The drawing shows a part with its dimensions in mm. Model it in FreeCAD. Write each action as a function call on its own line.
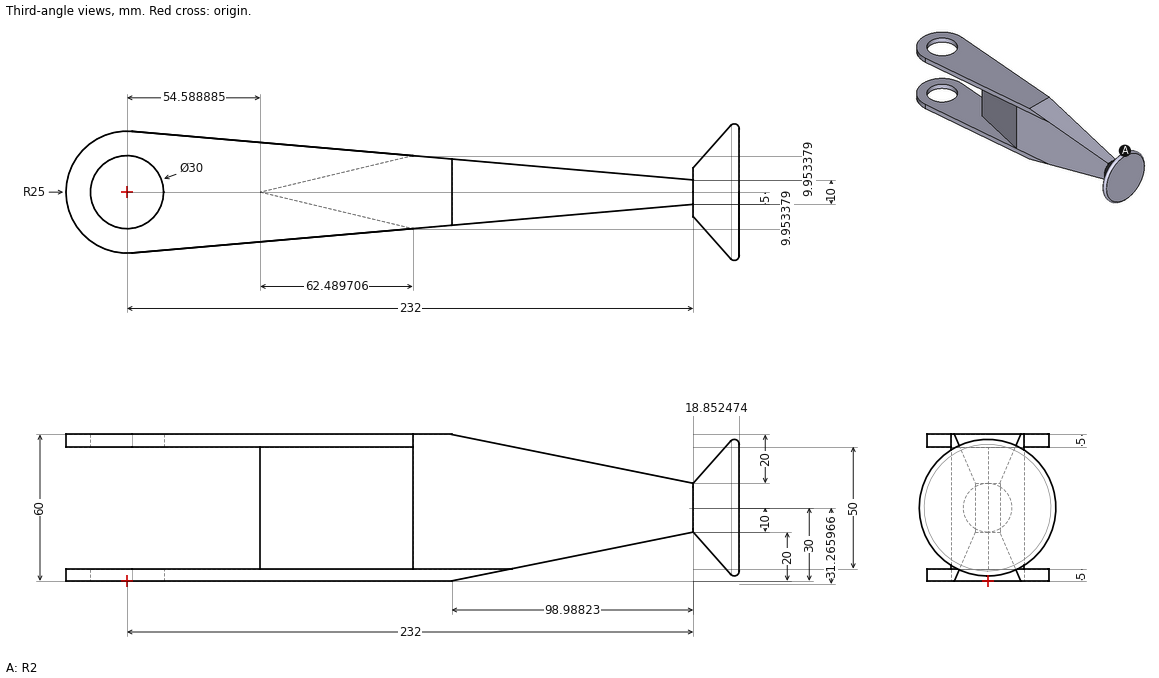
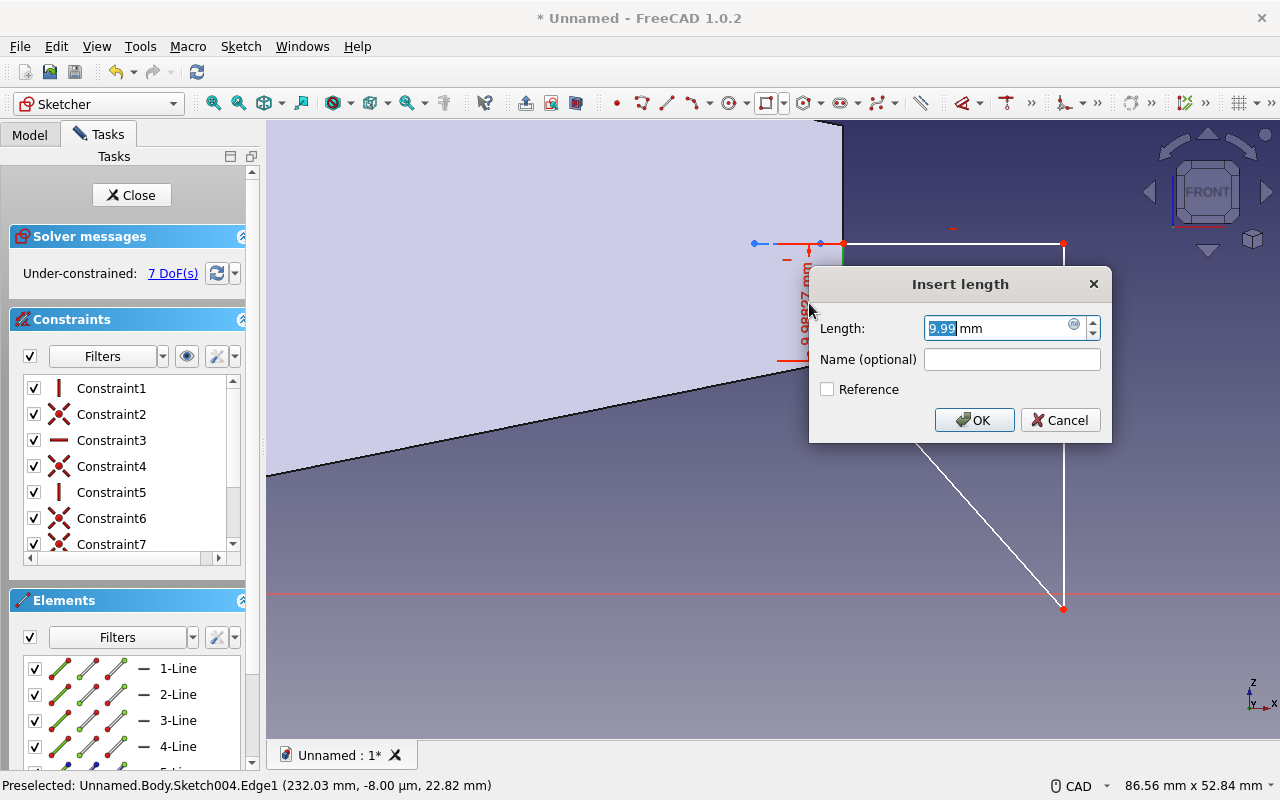
text(10)
key(Return)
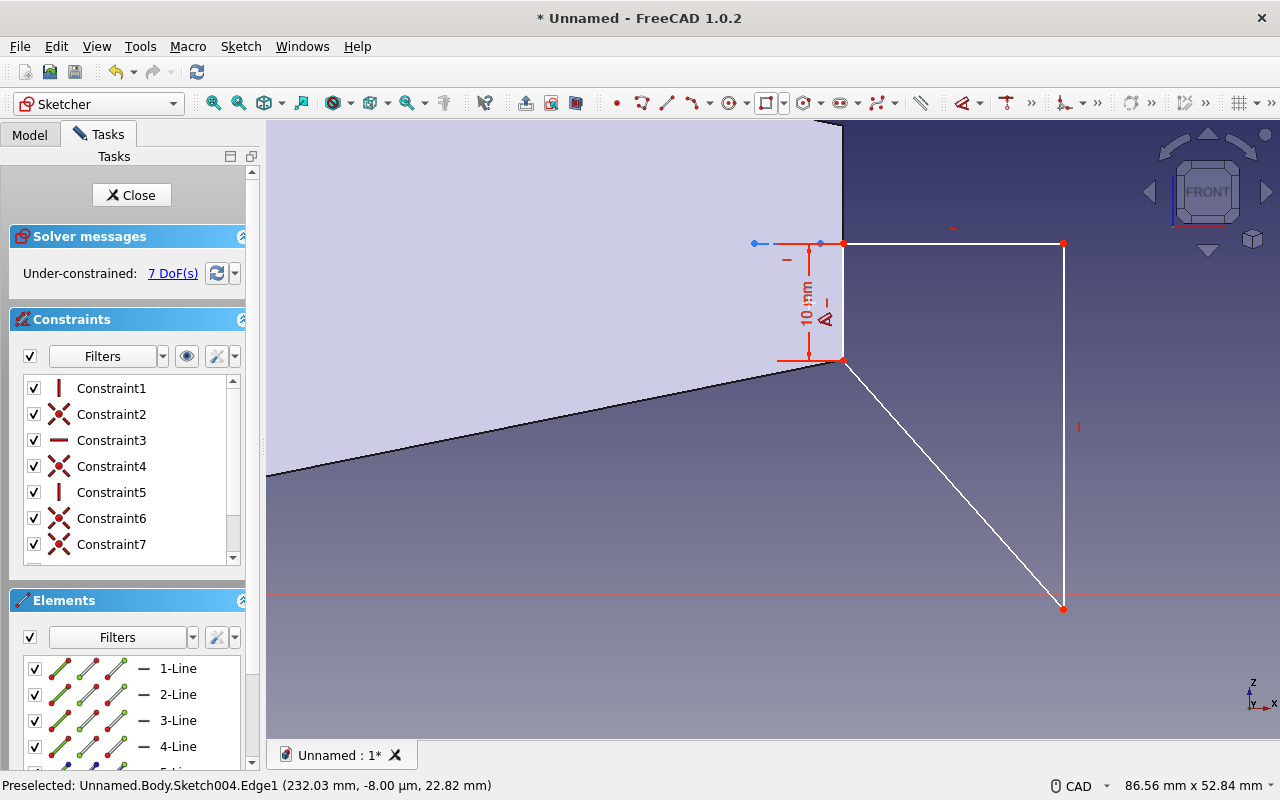
click(843, 361)
click(877, 478)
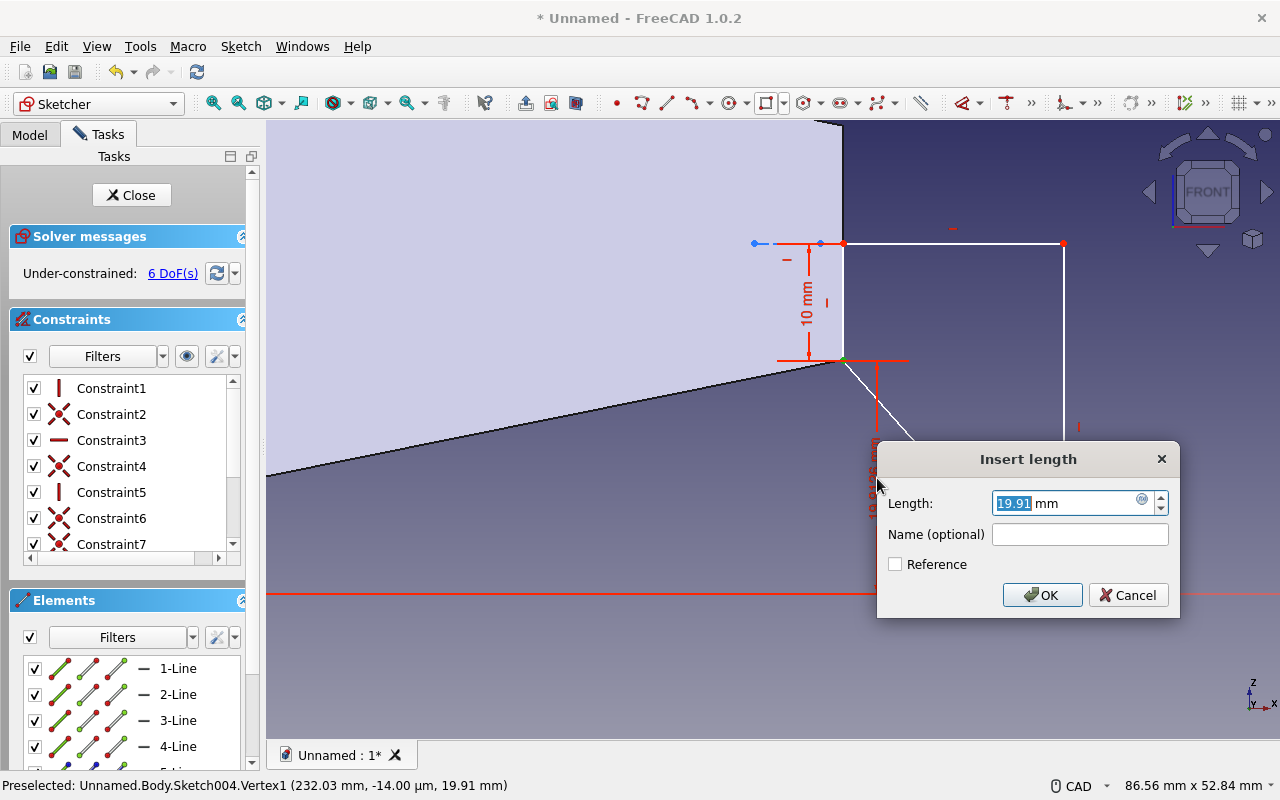
text(20)
key(Return)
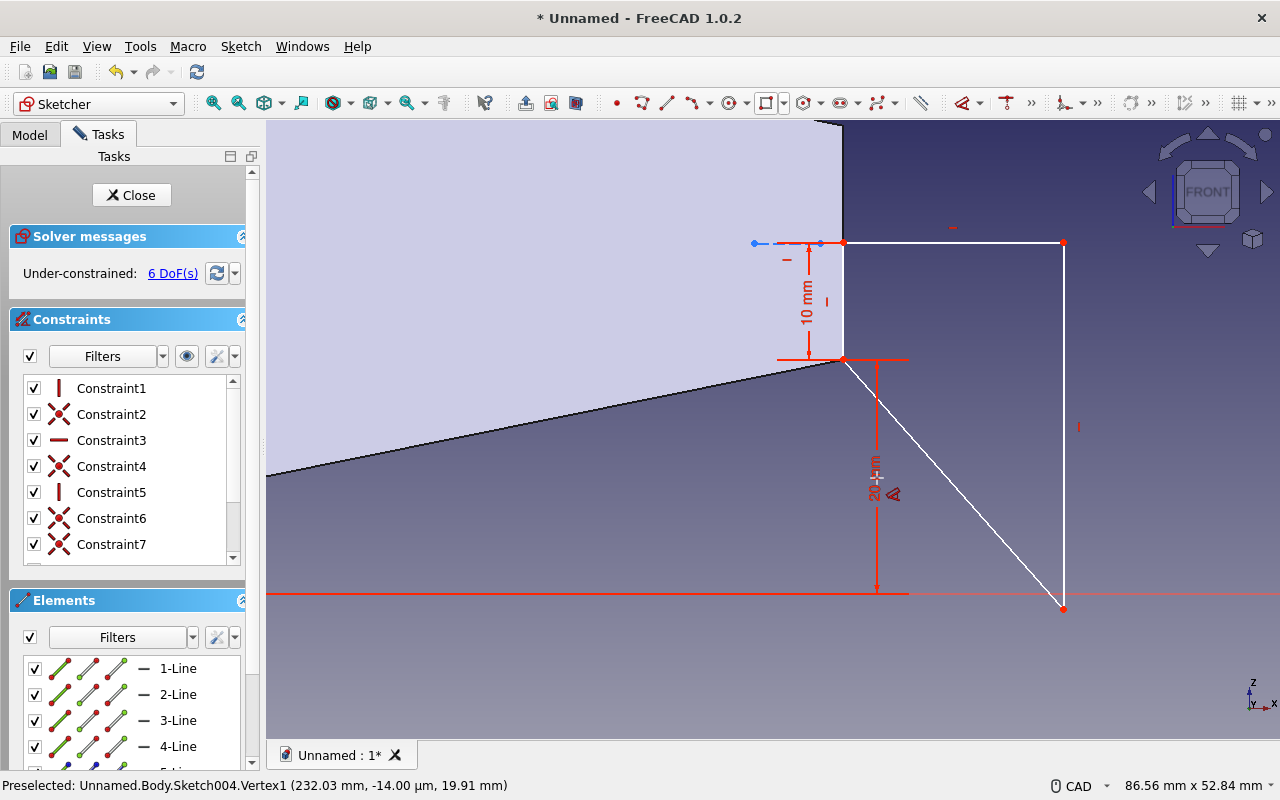
click(821, 244)
click(855, 419)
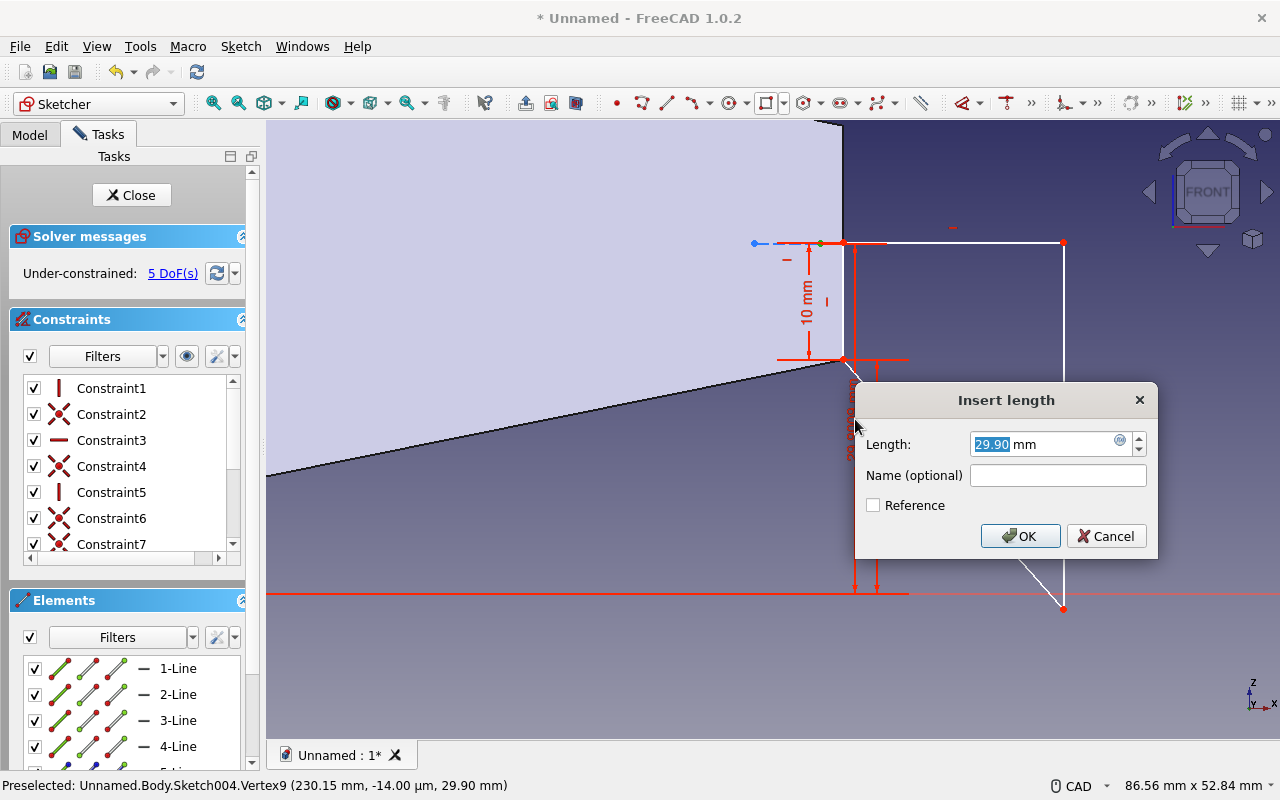
text(30)
key(Return)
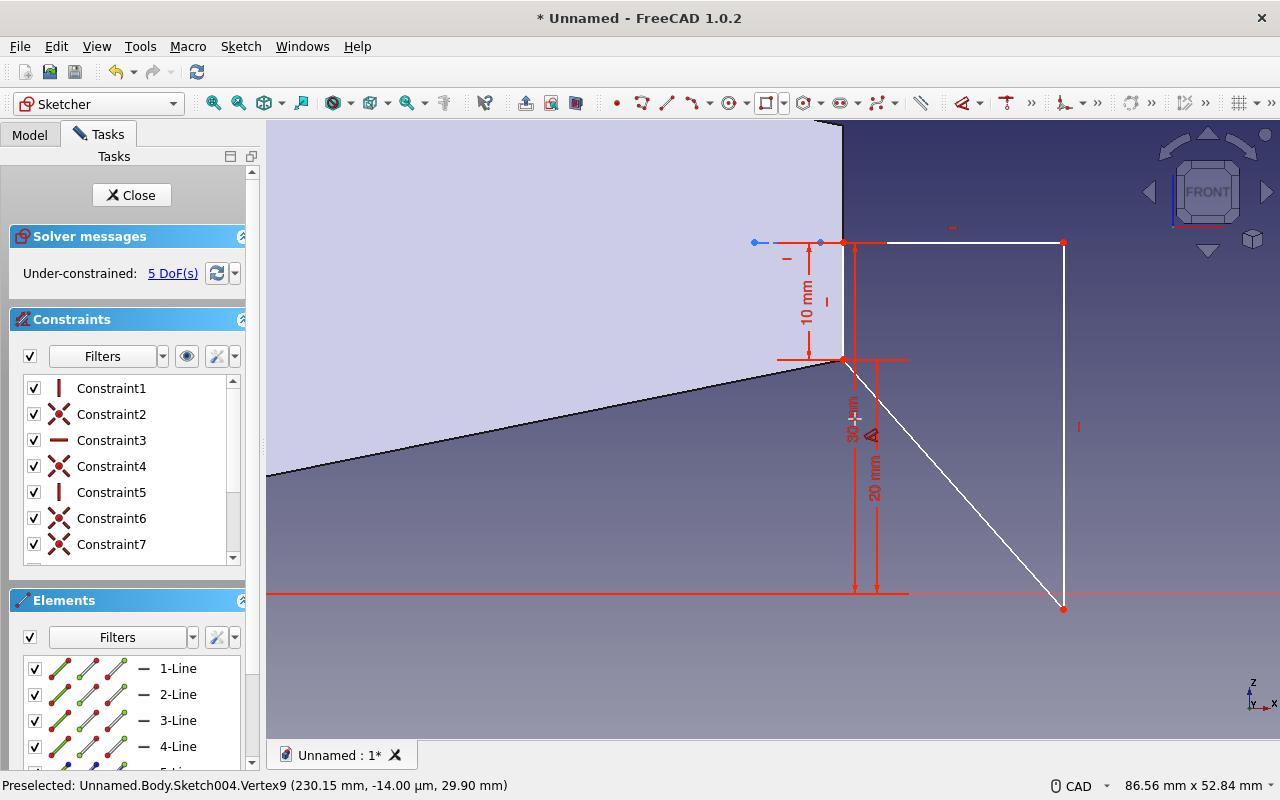
click(843, 360)
click(568, 628)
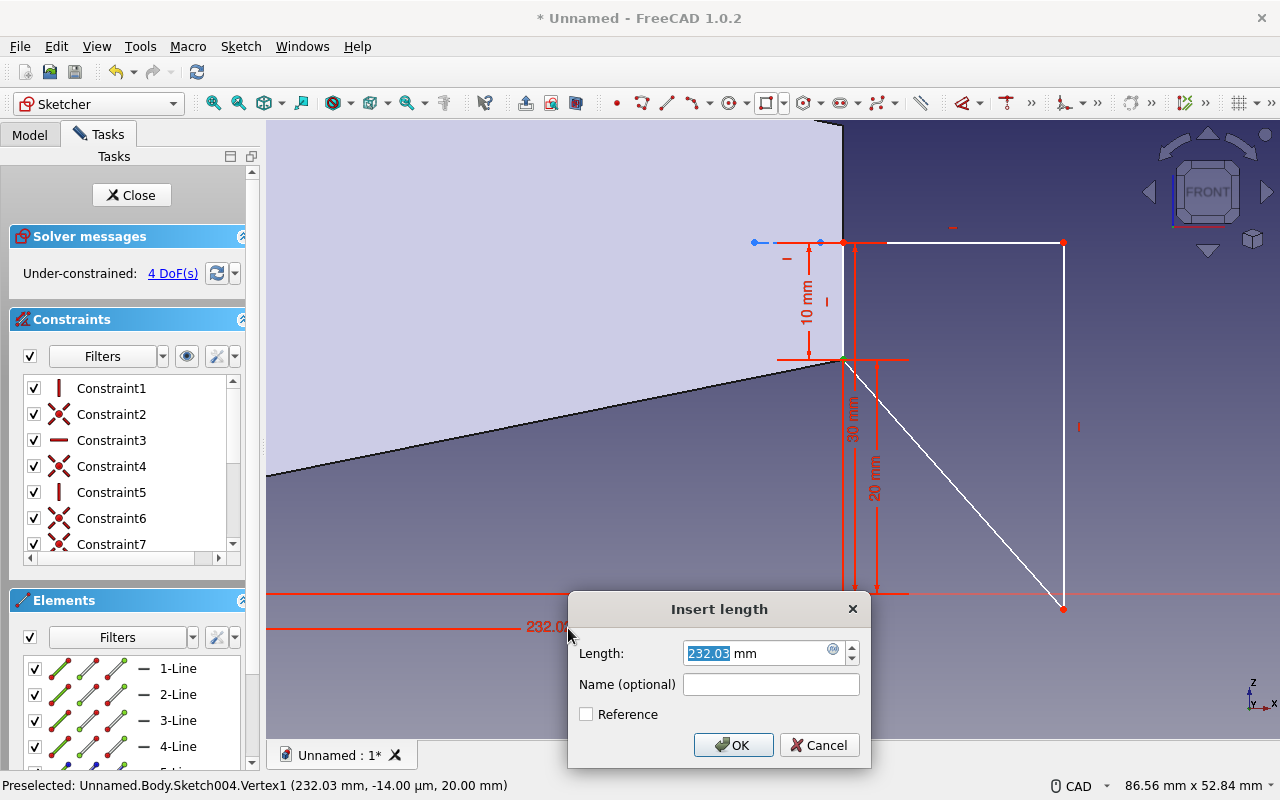
text(232)
key(Return)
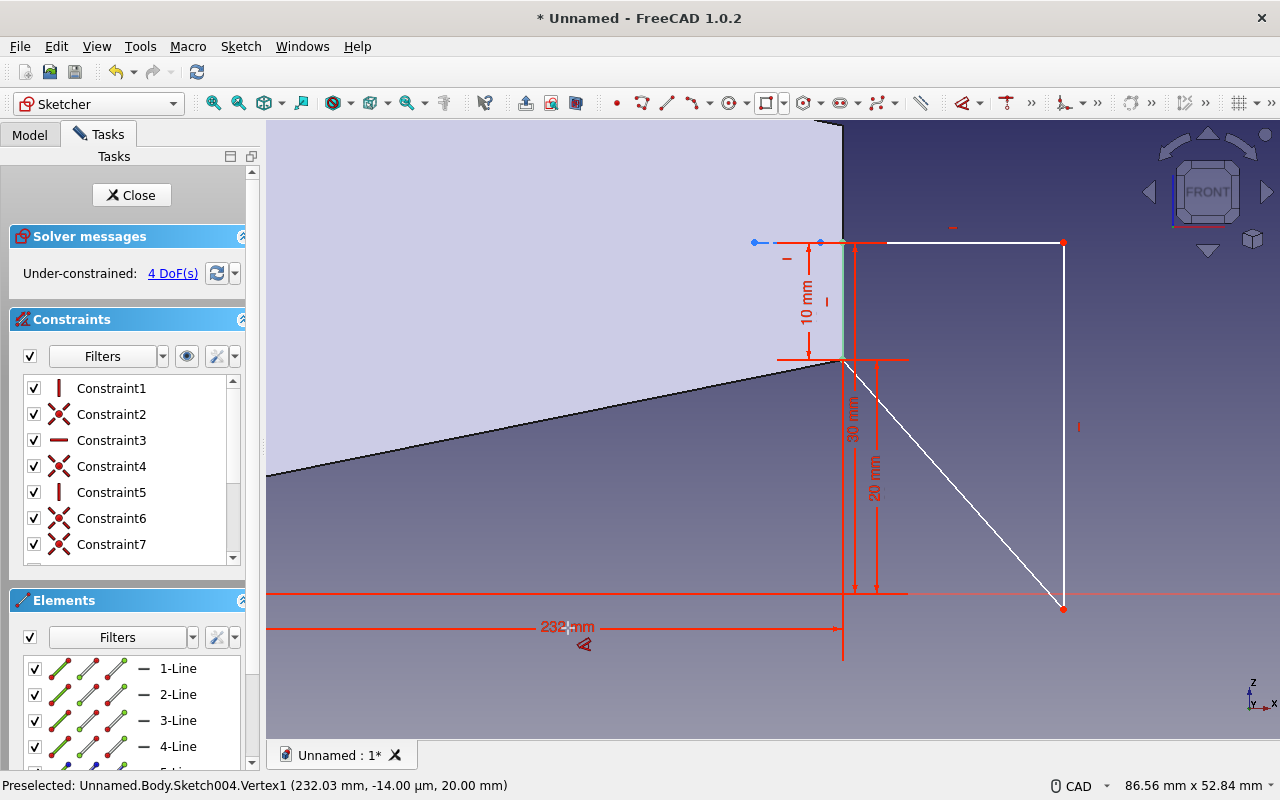
click(909, 243)
click(953, 209)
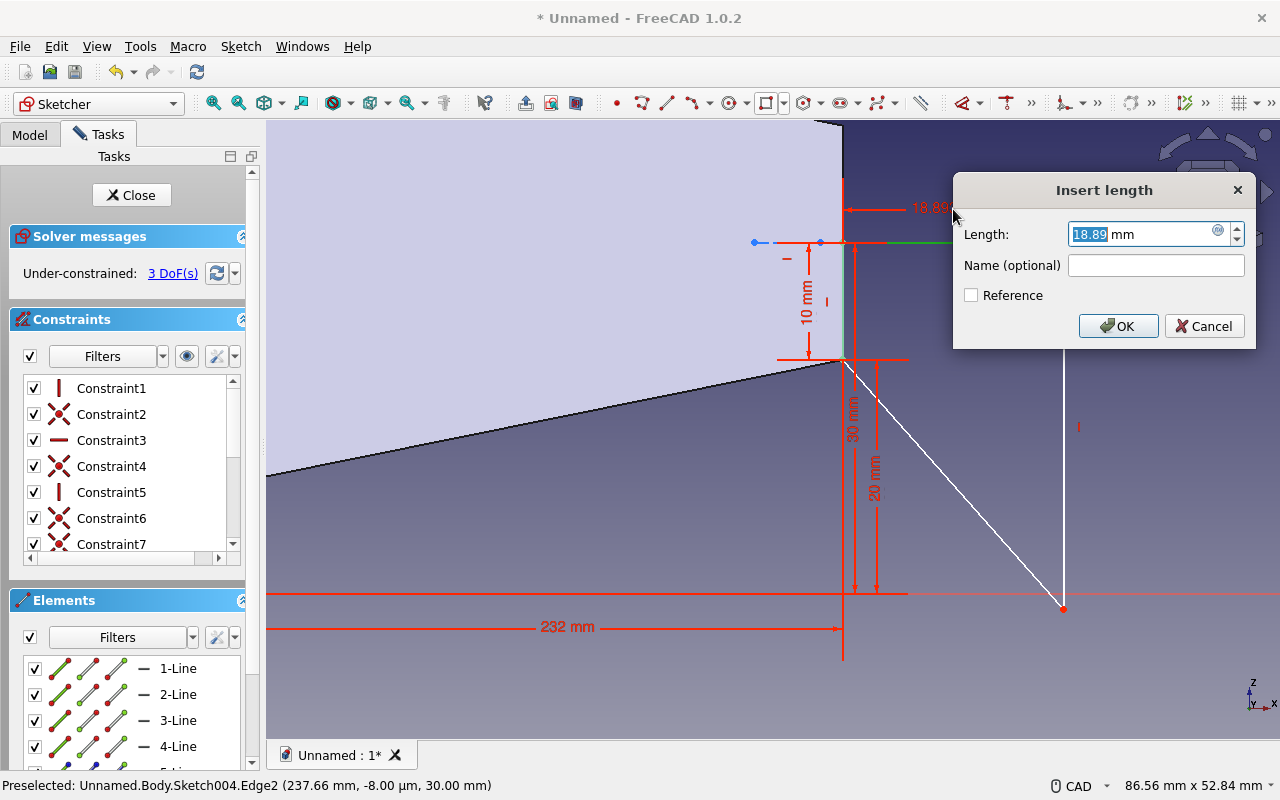
text(18.852474)
key(Return)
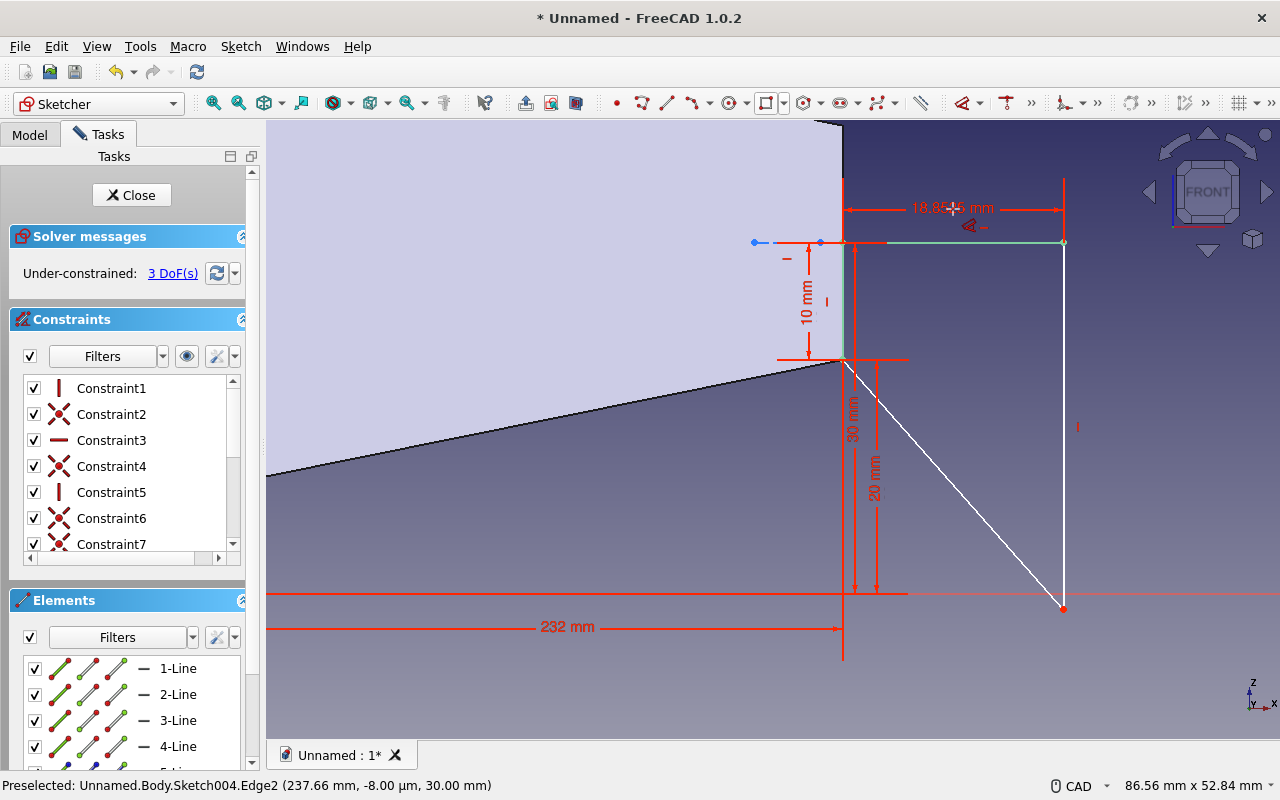
click(1064, 353)
click(1098, 426)